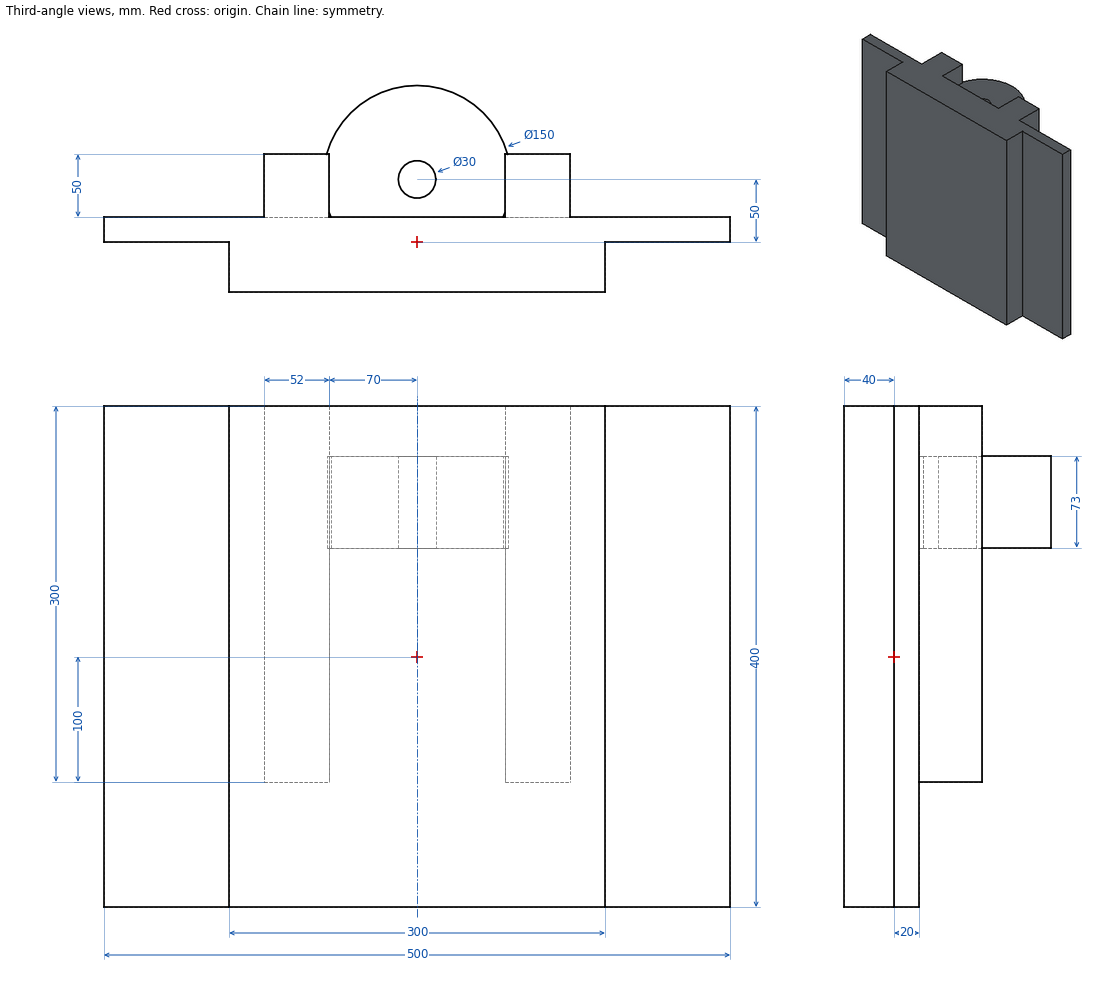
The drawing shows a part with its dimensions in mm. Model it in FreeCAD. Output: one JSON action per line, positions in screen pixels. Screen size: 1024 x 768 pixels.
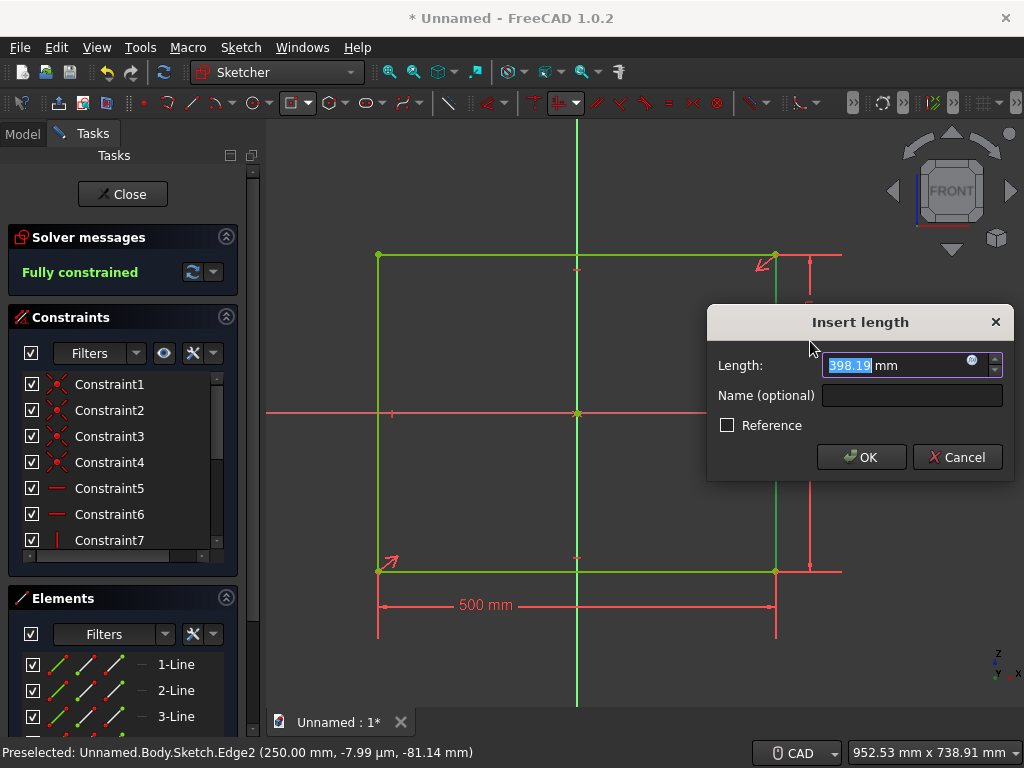
{"action": "type", "text": "400"}
{"action": "key", "text": "Return"}
{"action": "key", "text": "Escape"}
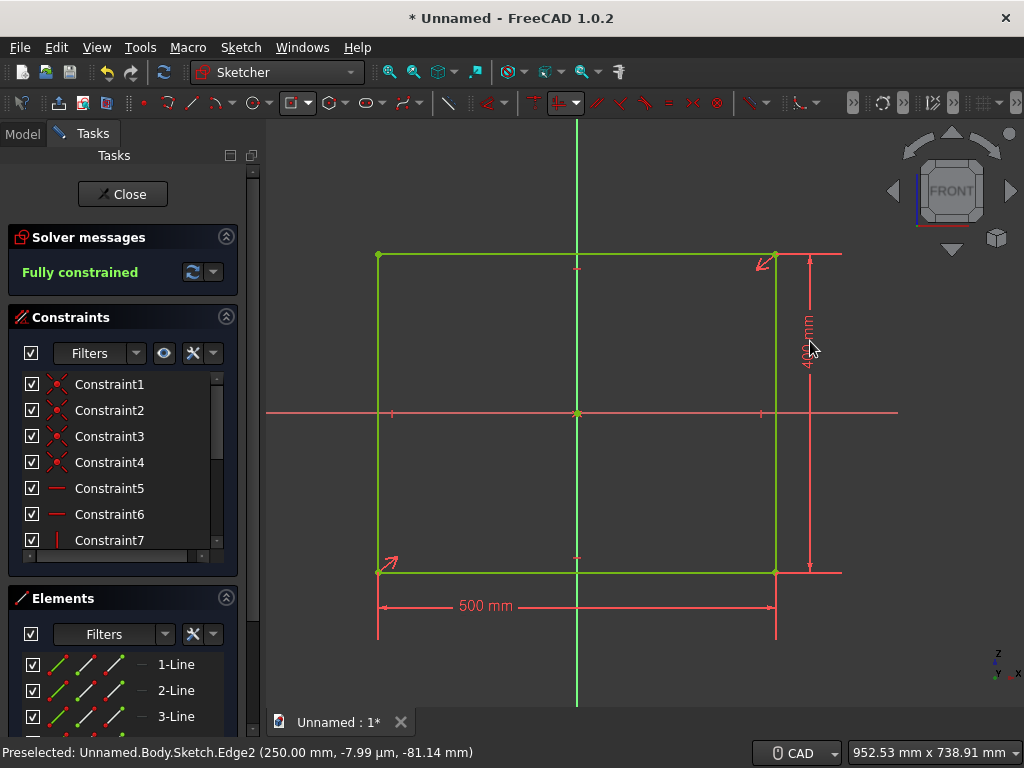
{"action": "left_click", "coordinate": [123, 194]}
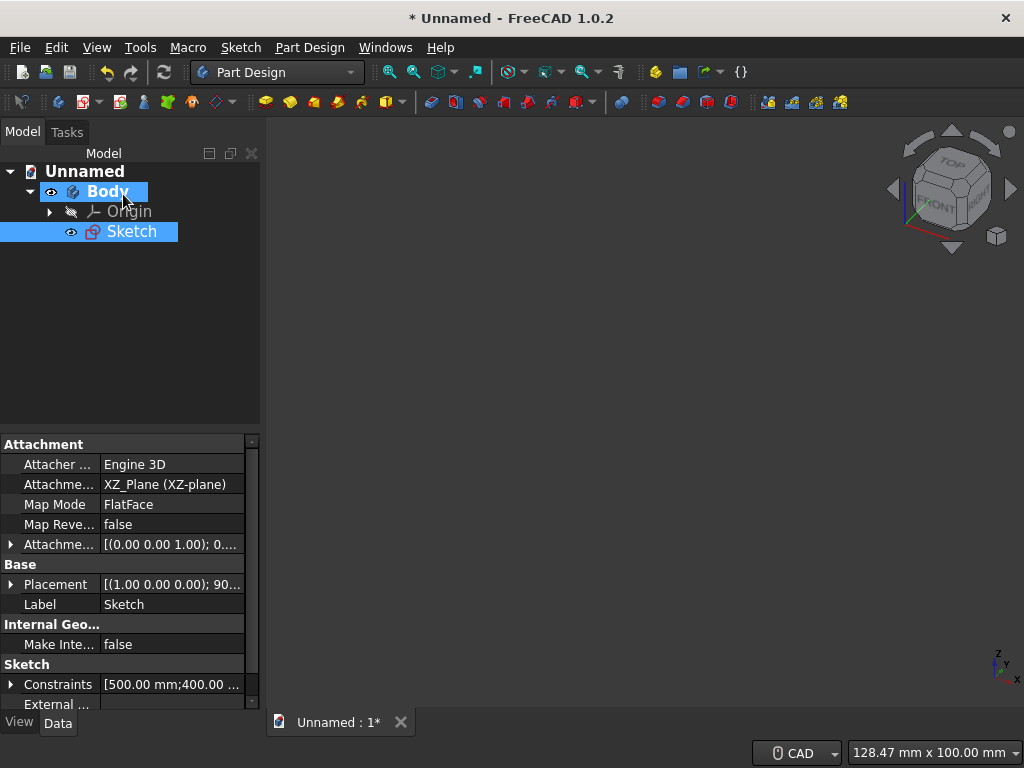
{"action": "left_click", "coordinate": [266, 102]}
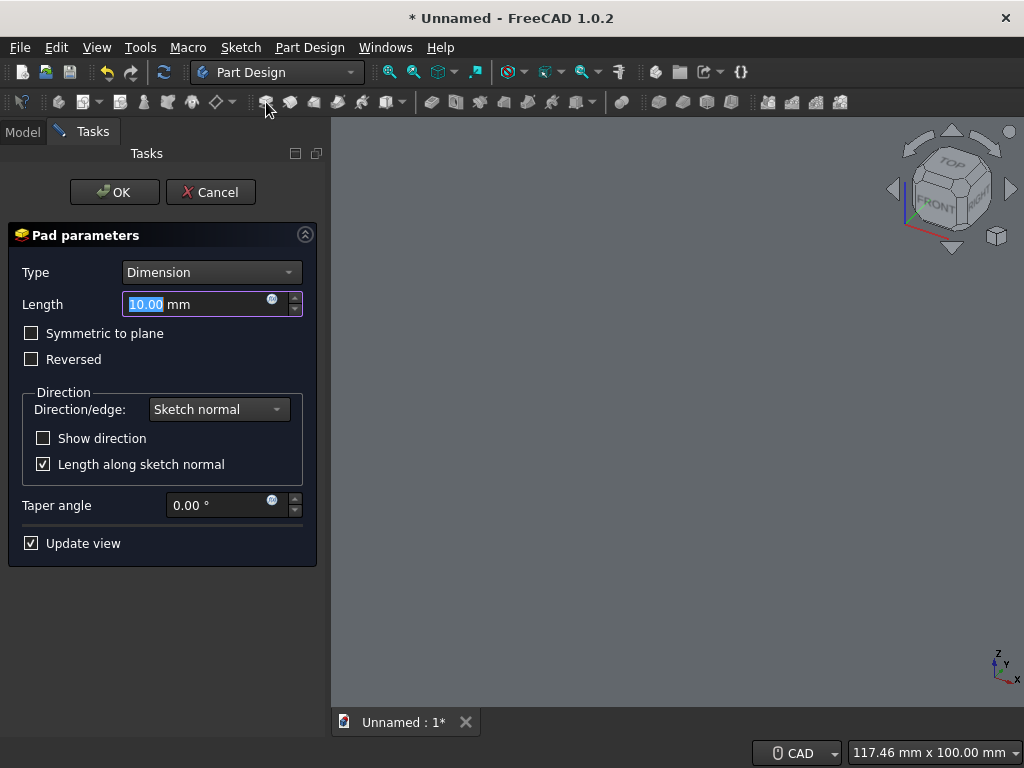
{"action": "type", "text": "20"}
{"action": "key", "text": "Tab"}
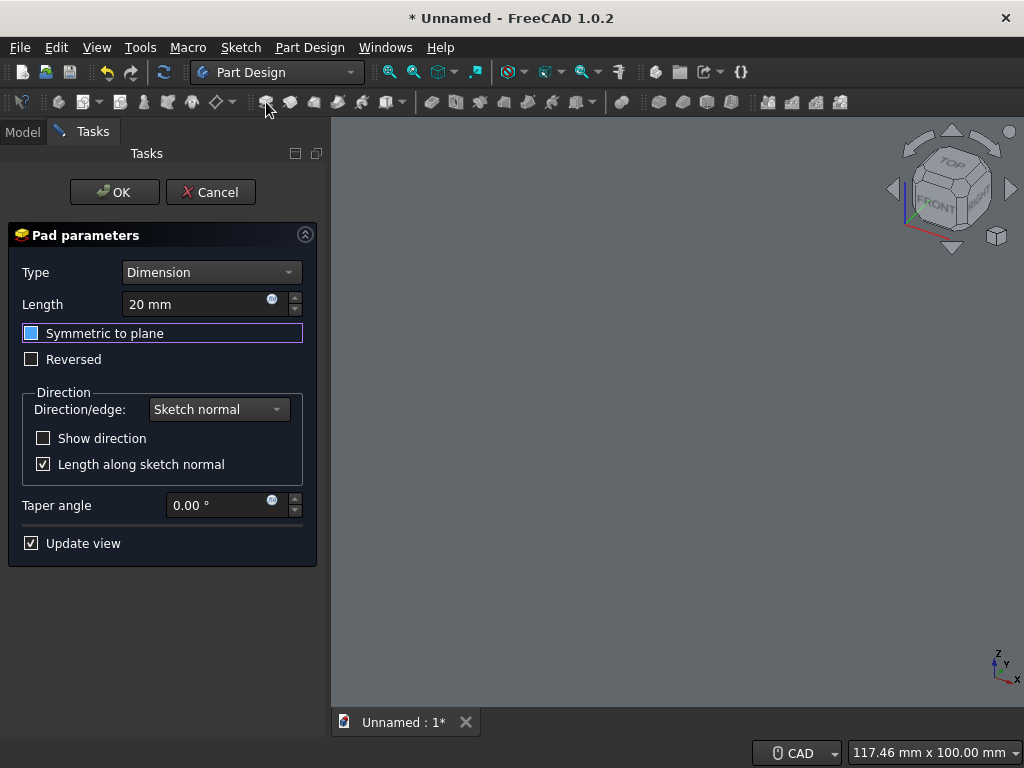
{"action": "left_click", "coordinate": [30, 359]}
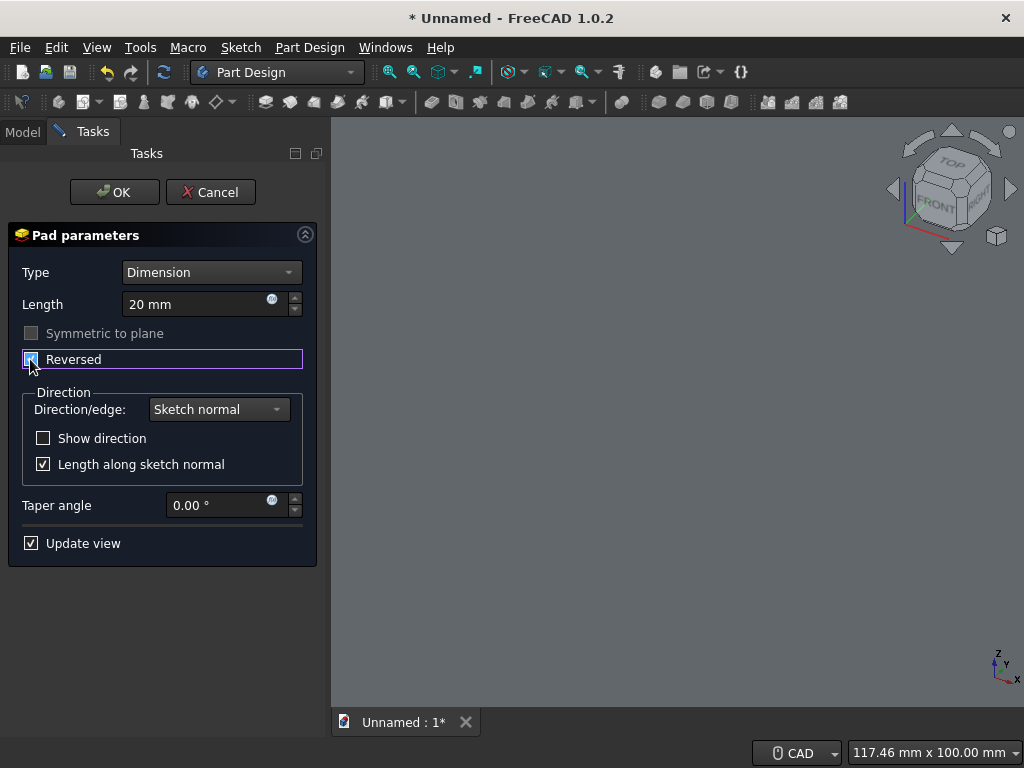
{"action": "left_click", "coordinate": [115, 192]}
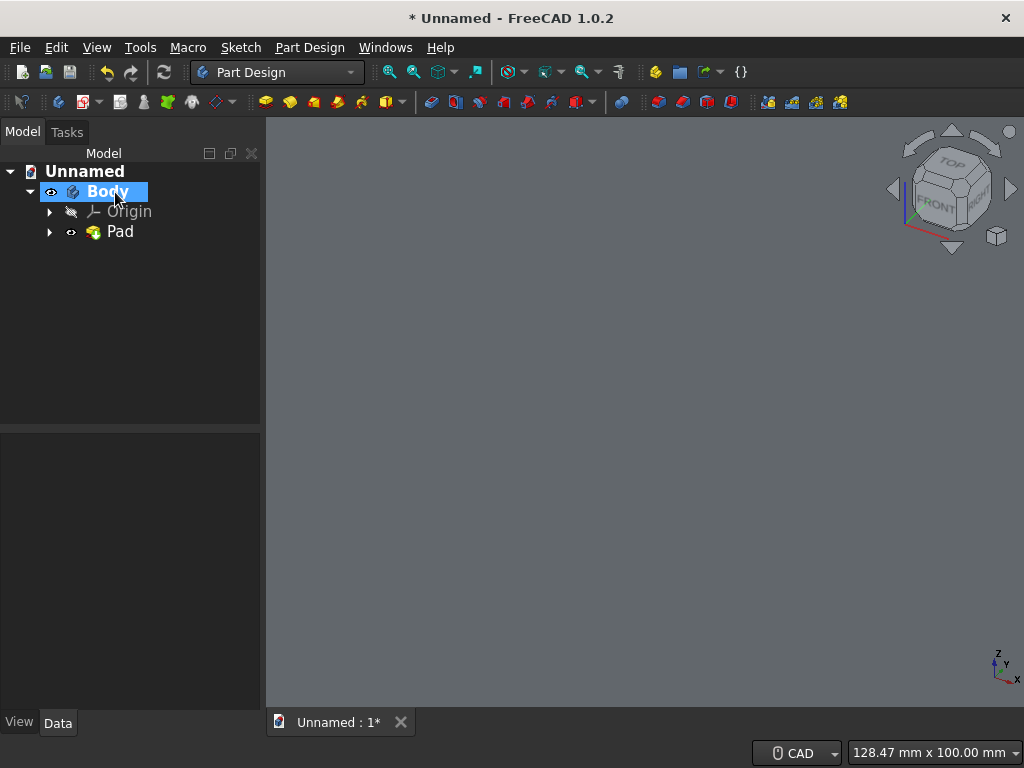
{"action": "key", "text": "v f"}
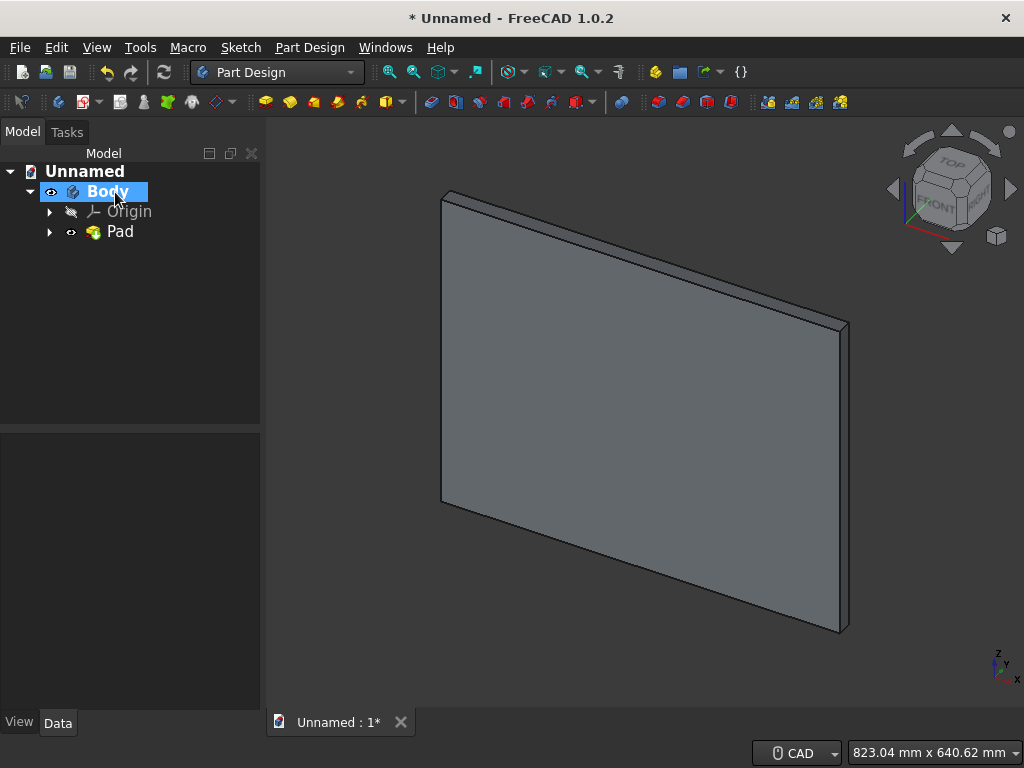
{"action": "key", "text": "4"}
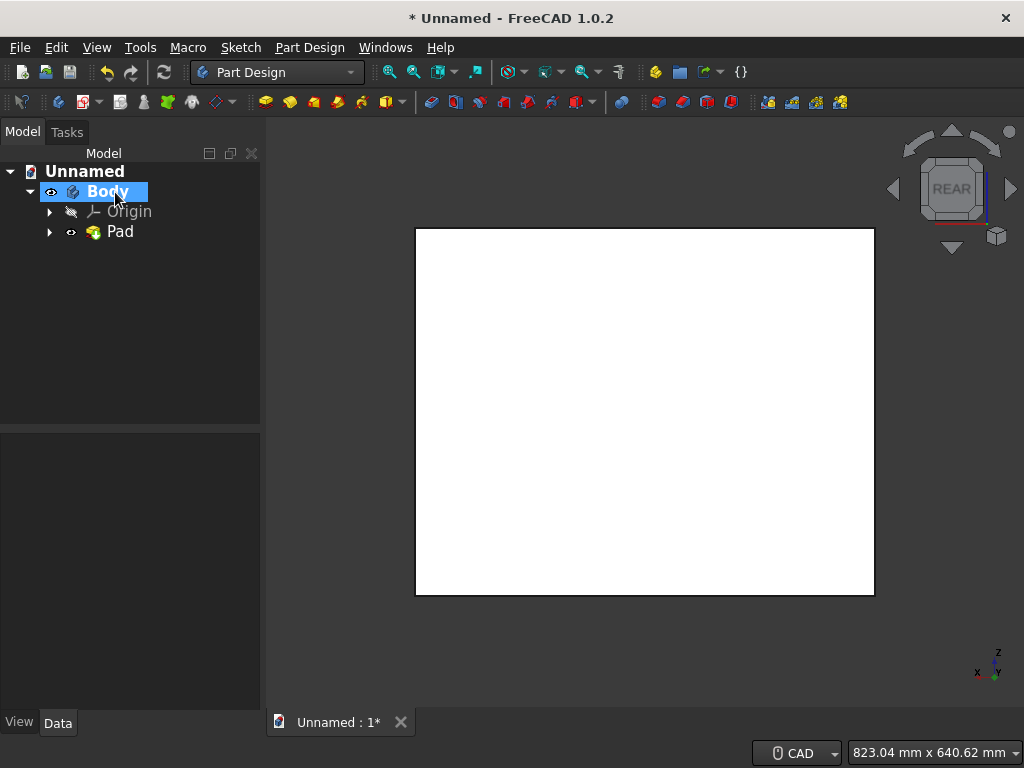
{"action": "left_click", "coordinate": [645, 411]}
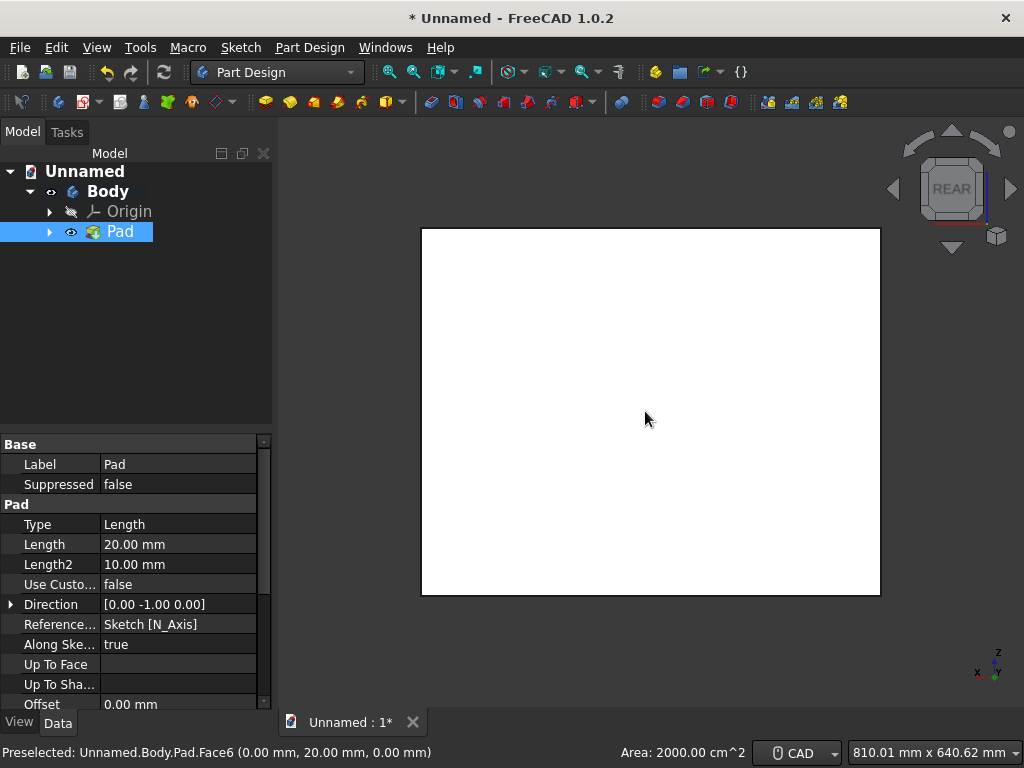
{"action": "left_click", "coordinate": [84, 102]}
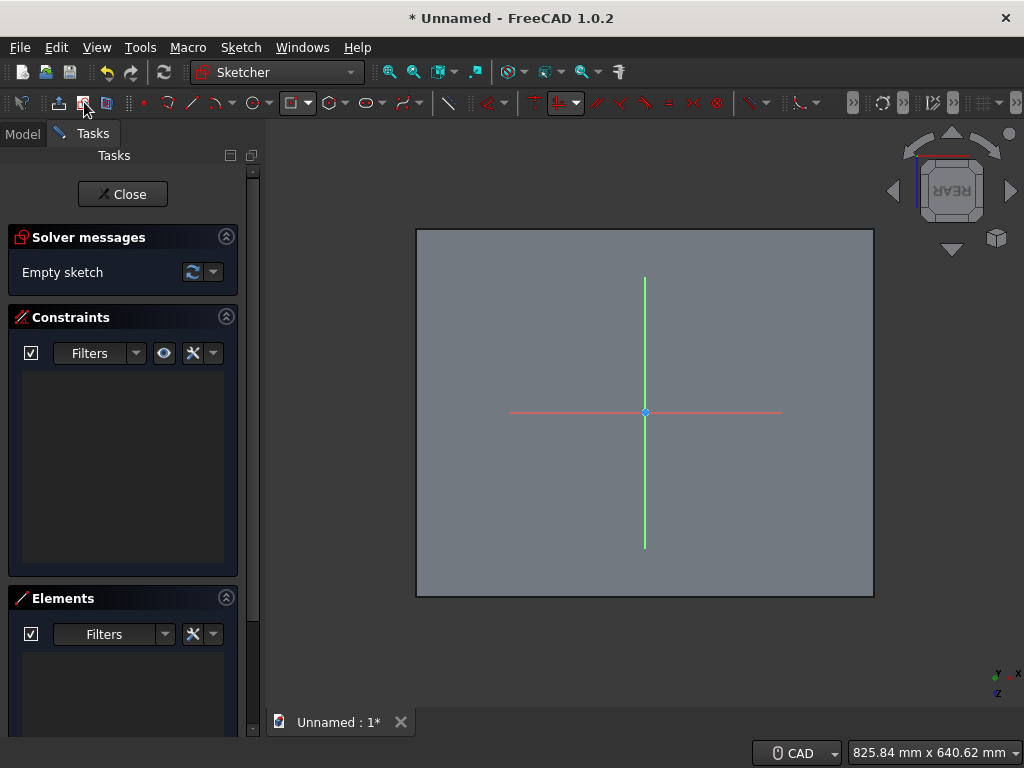
{"action": "scroll", "coordinate": [784, 552], "scroll_direction": "up", "scroll_amount": 2}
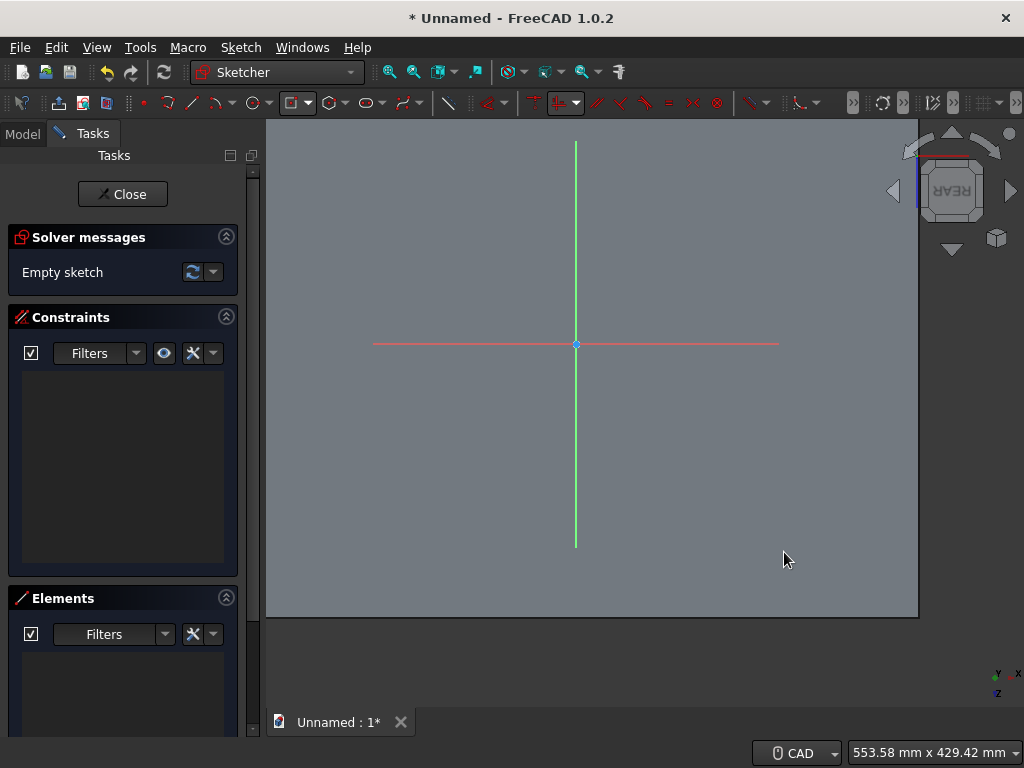
{"action": "left_click", "coordinate": [310, 104]}